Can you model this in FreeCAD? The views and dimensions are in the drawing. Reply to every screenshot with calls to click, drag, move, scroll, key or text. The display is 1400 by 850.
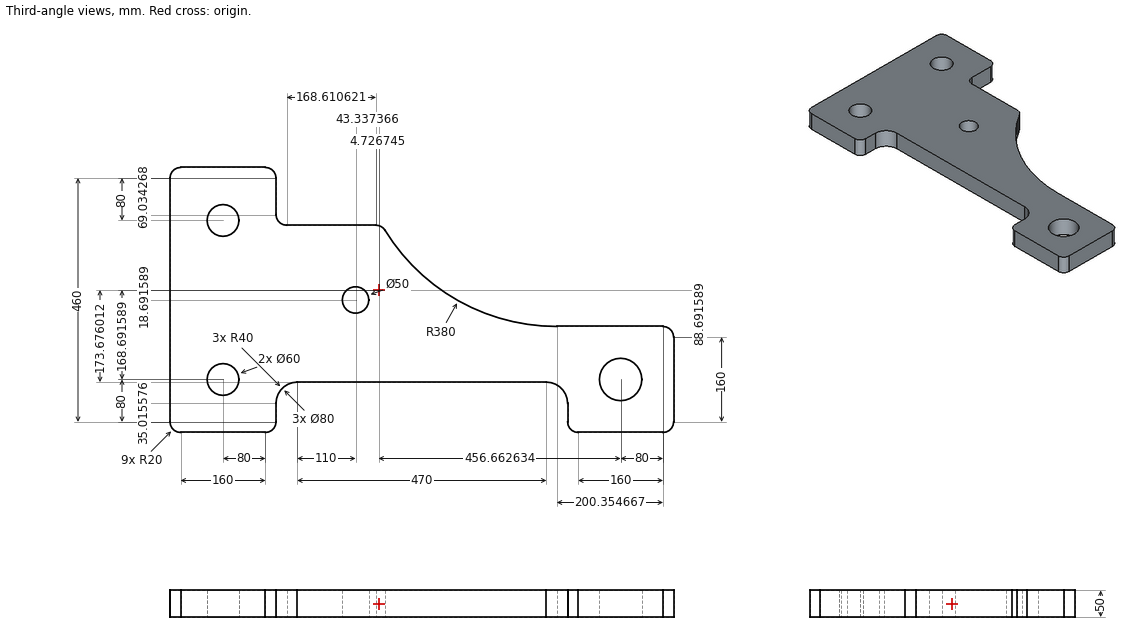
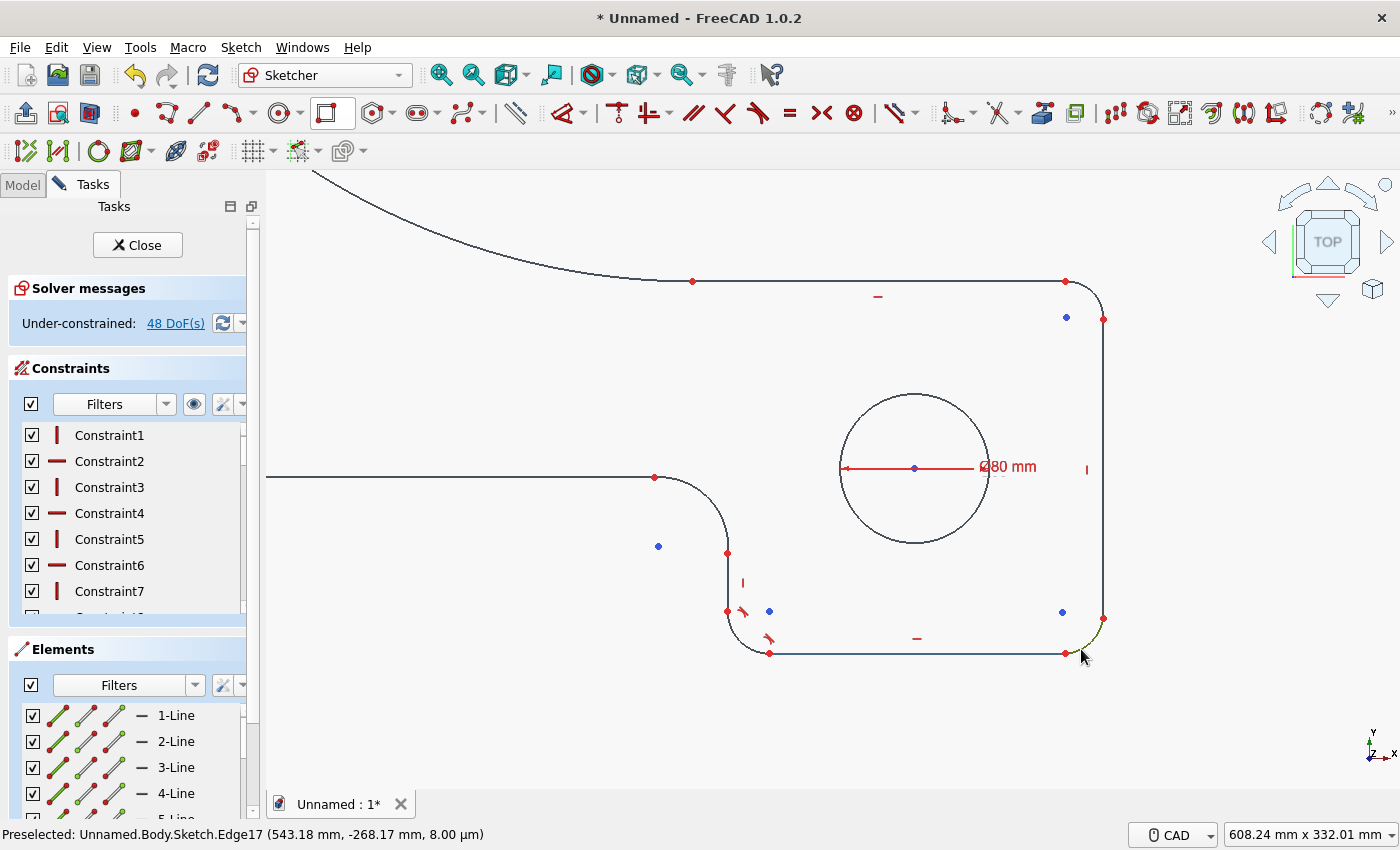
click(758, 114)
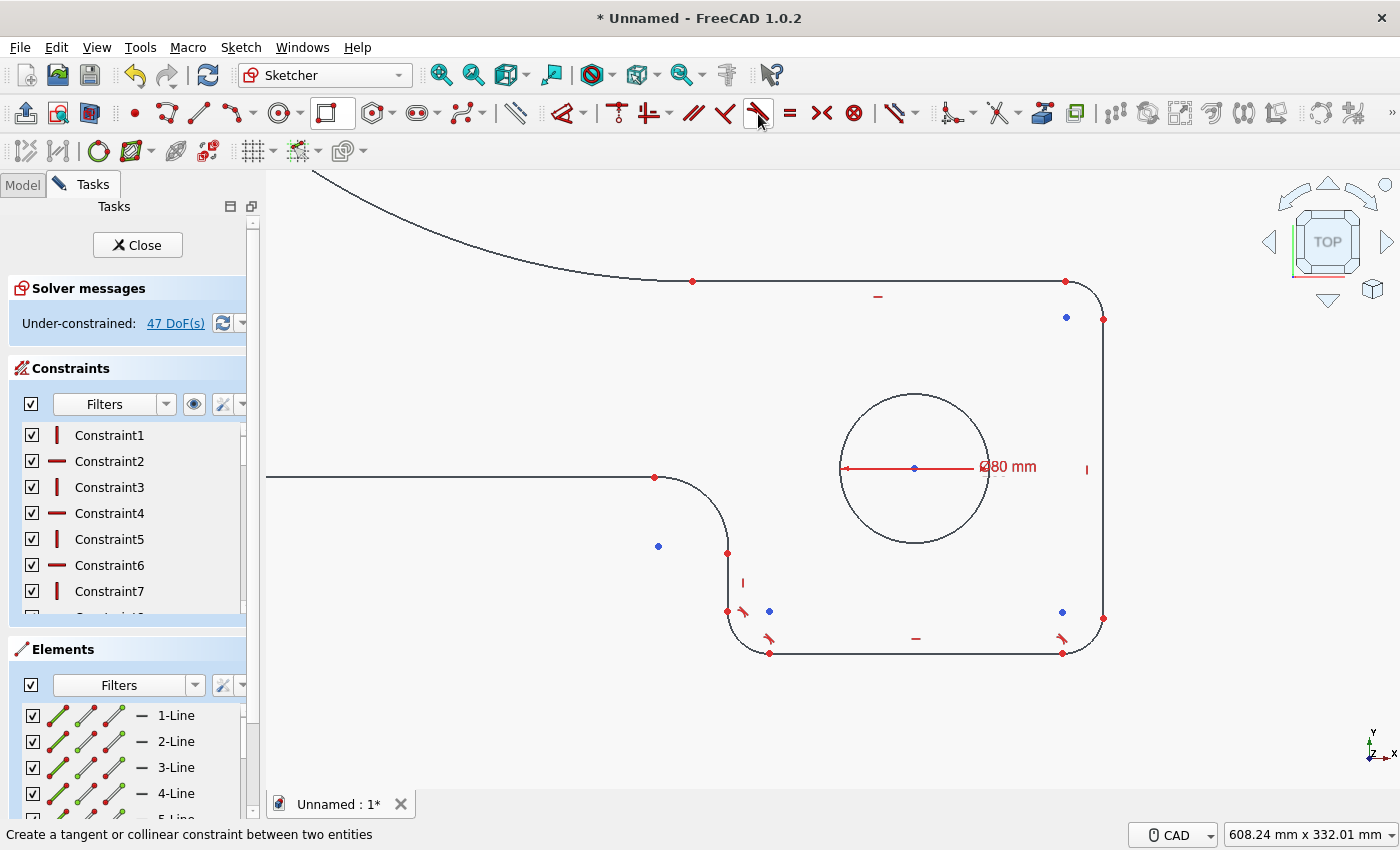
click(1103, 529)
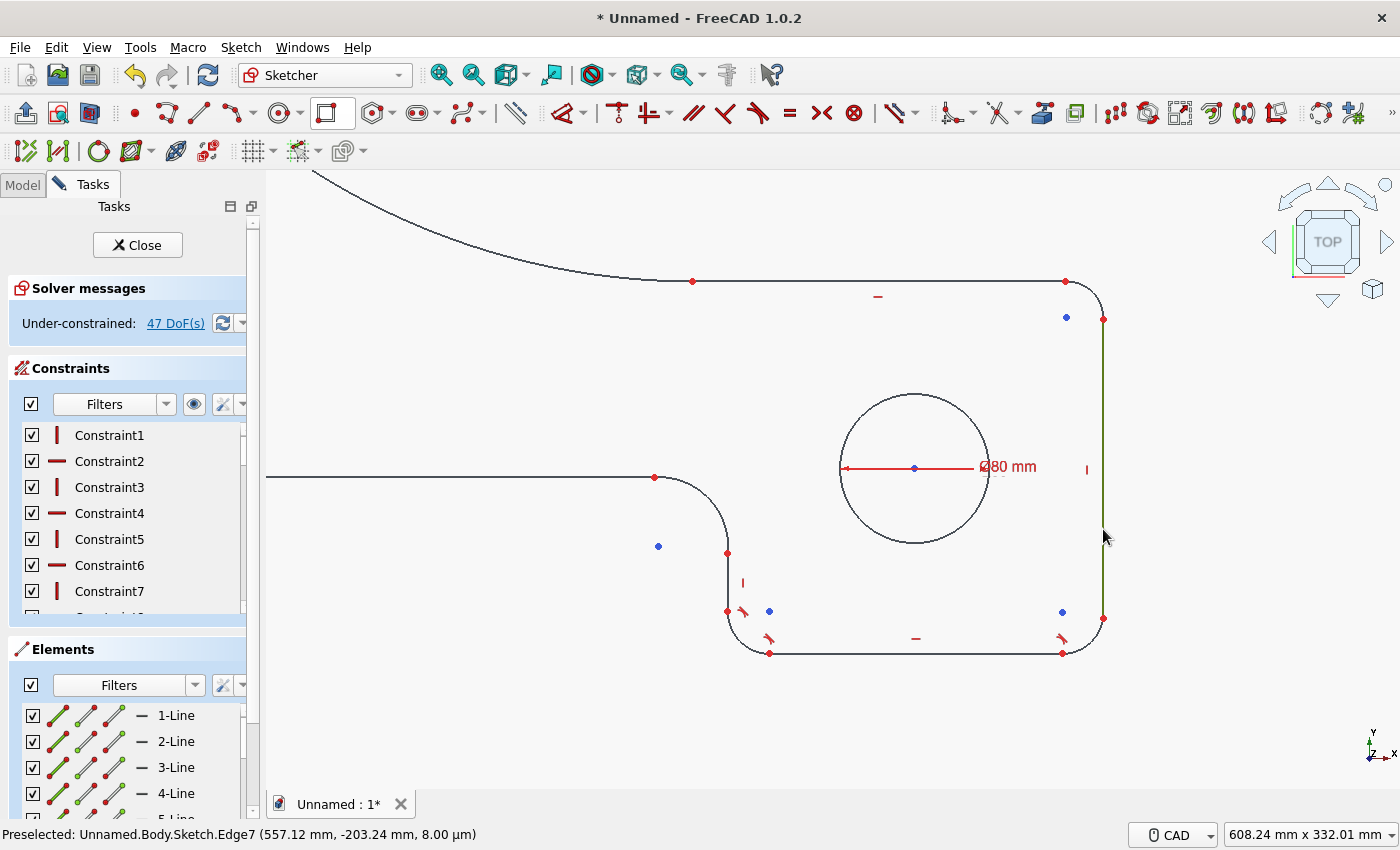
click(1079, 650)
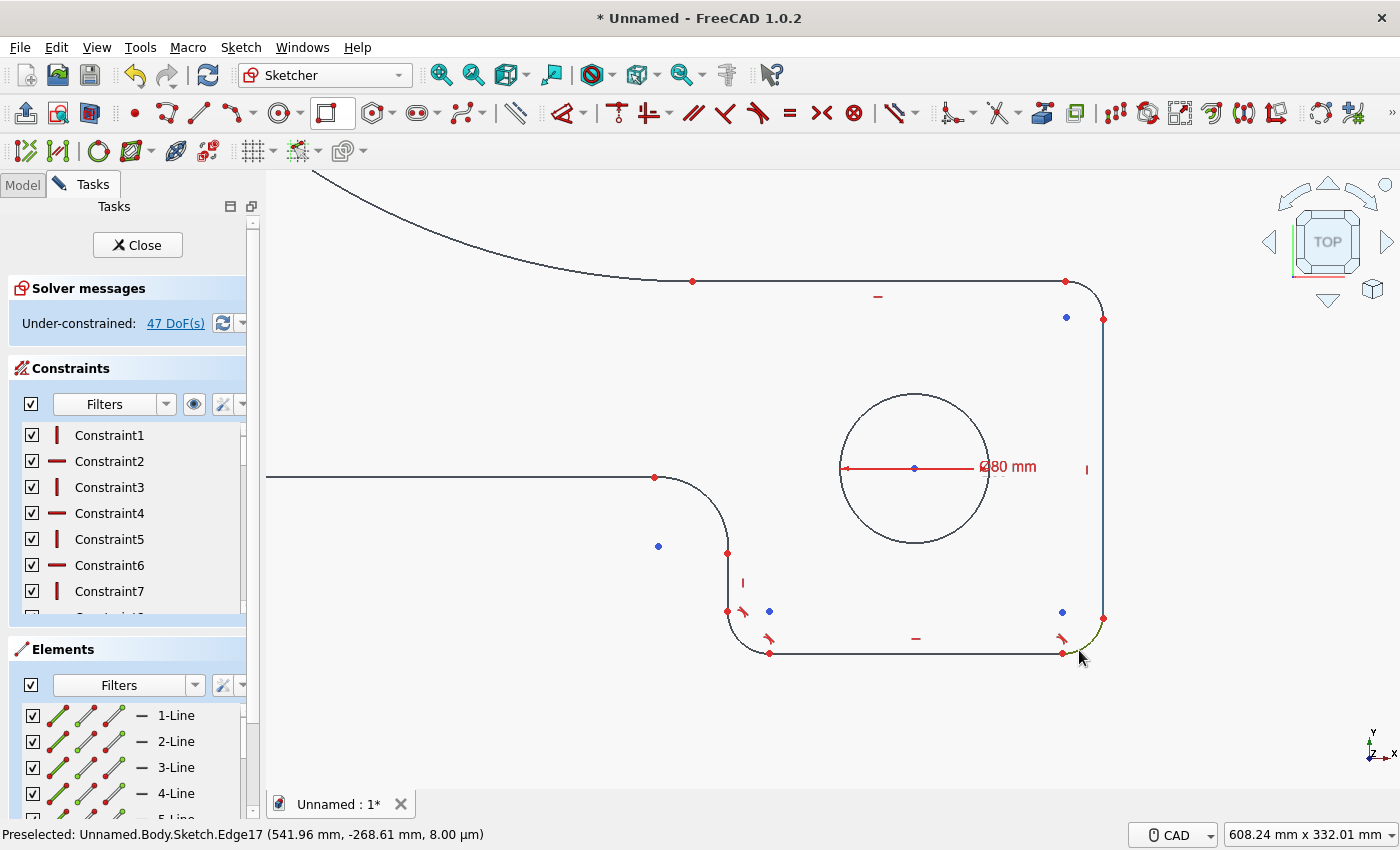
click(758, 114)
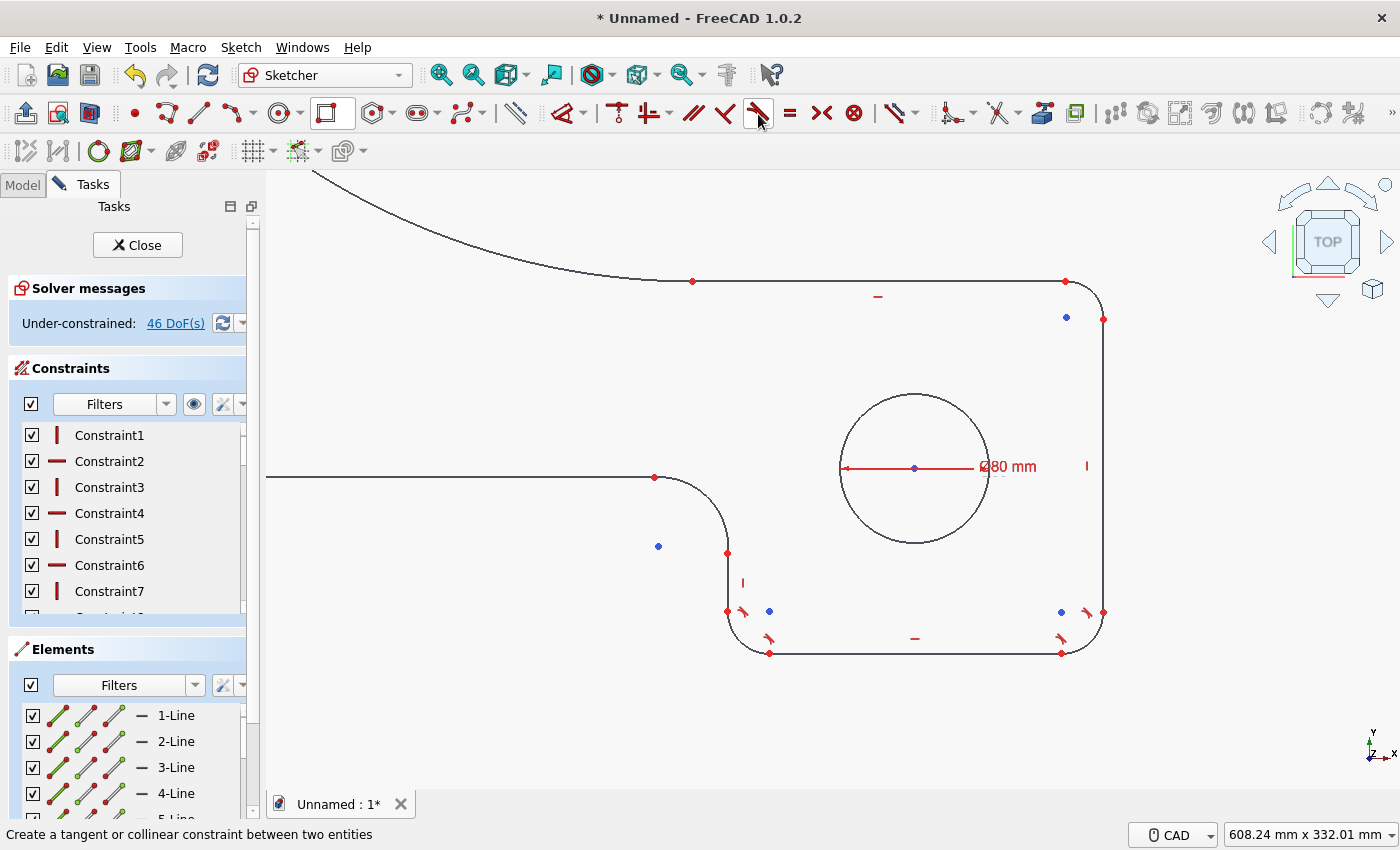
click(1103, 524)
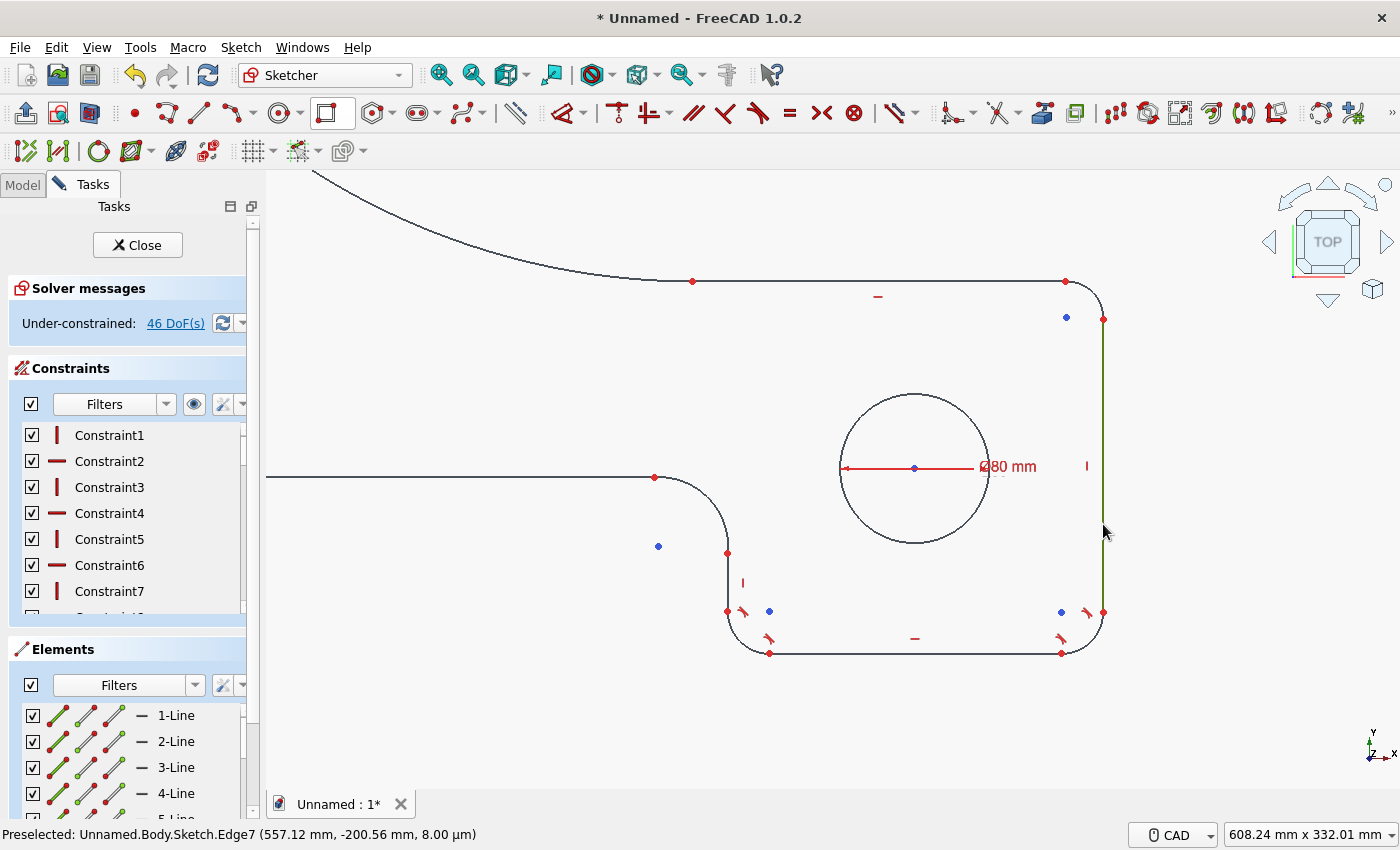
click(1100, 302)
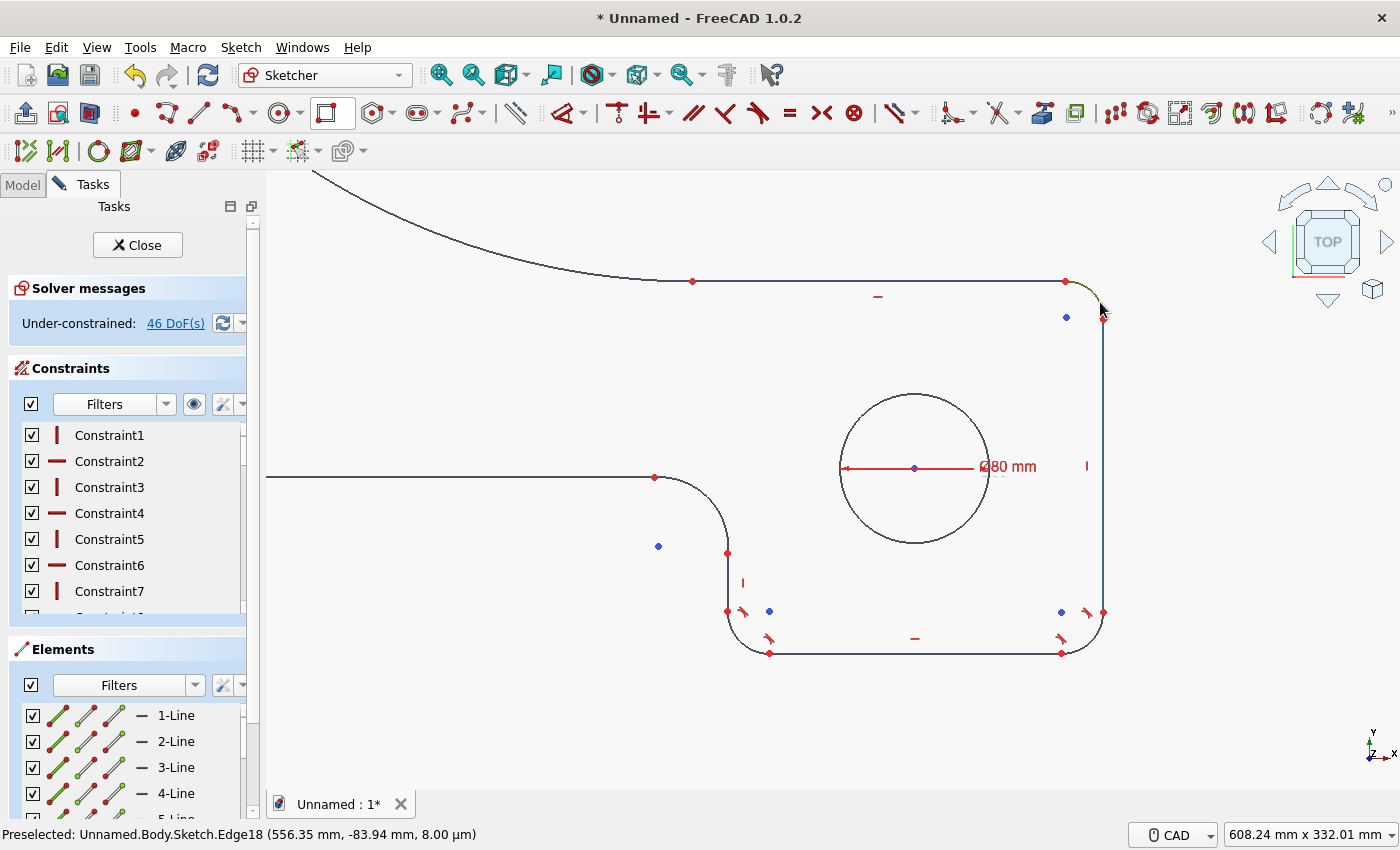
click(758, 114)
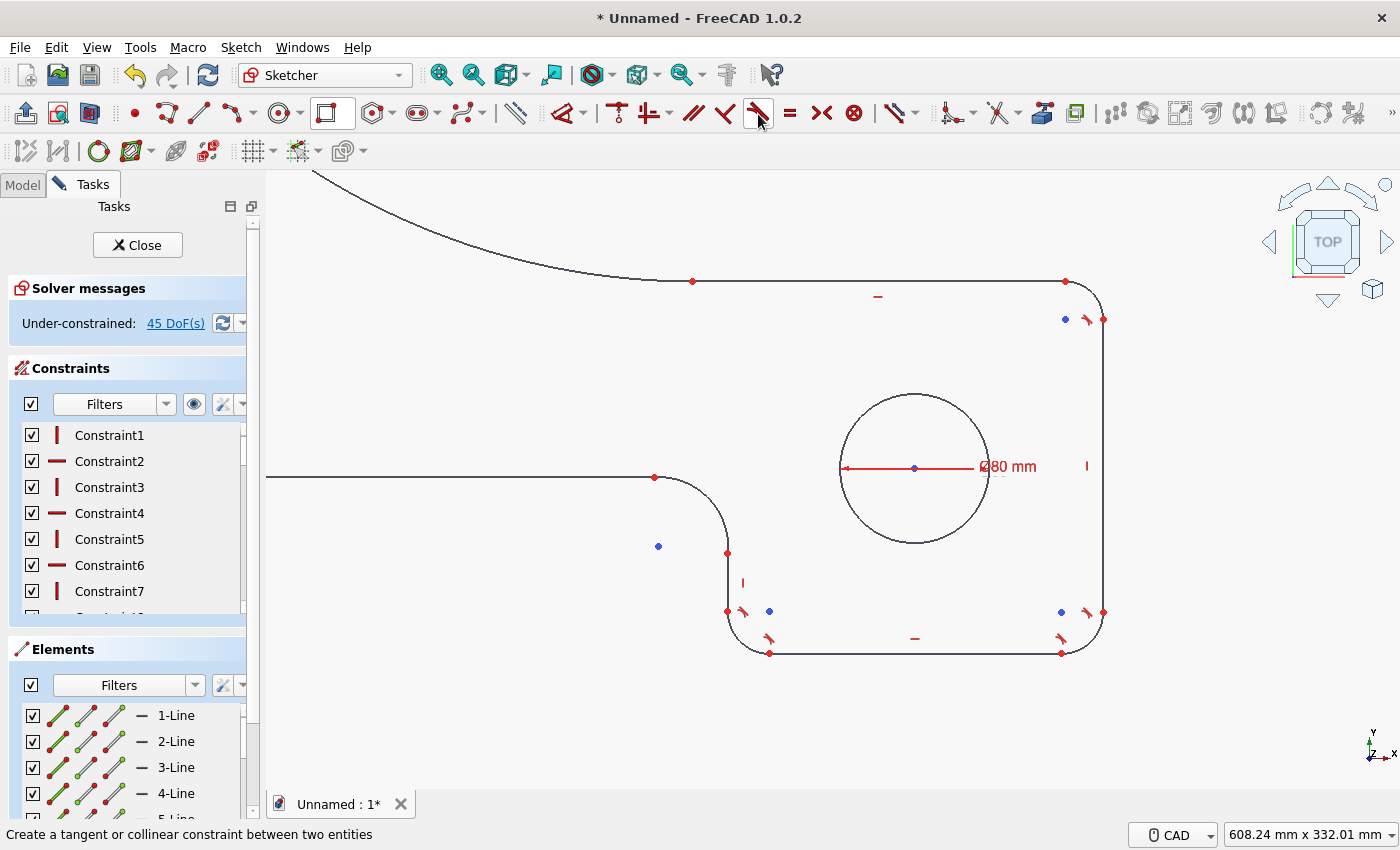
click(953, 281)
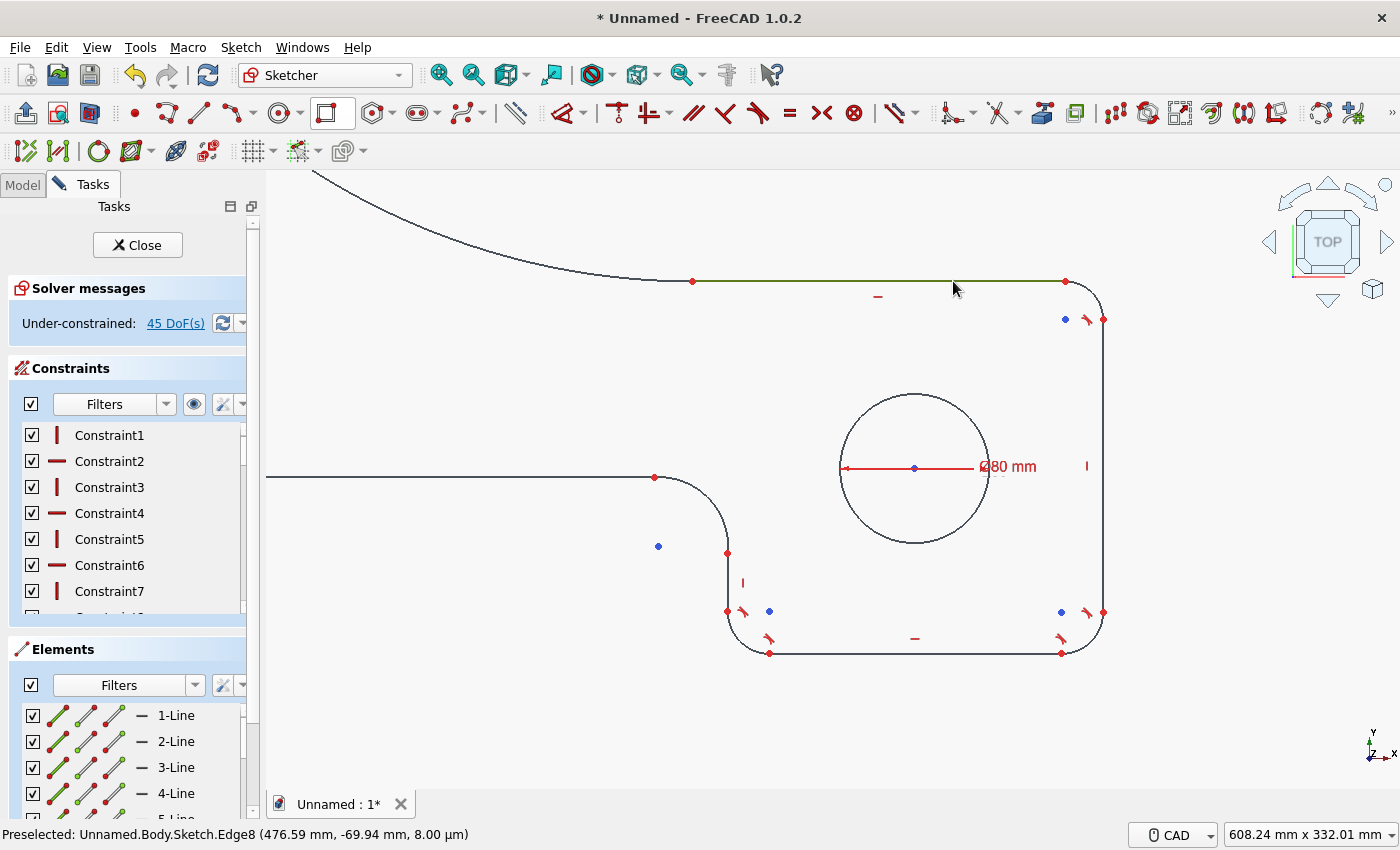
click(1099, 302)